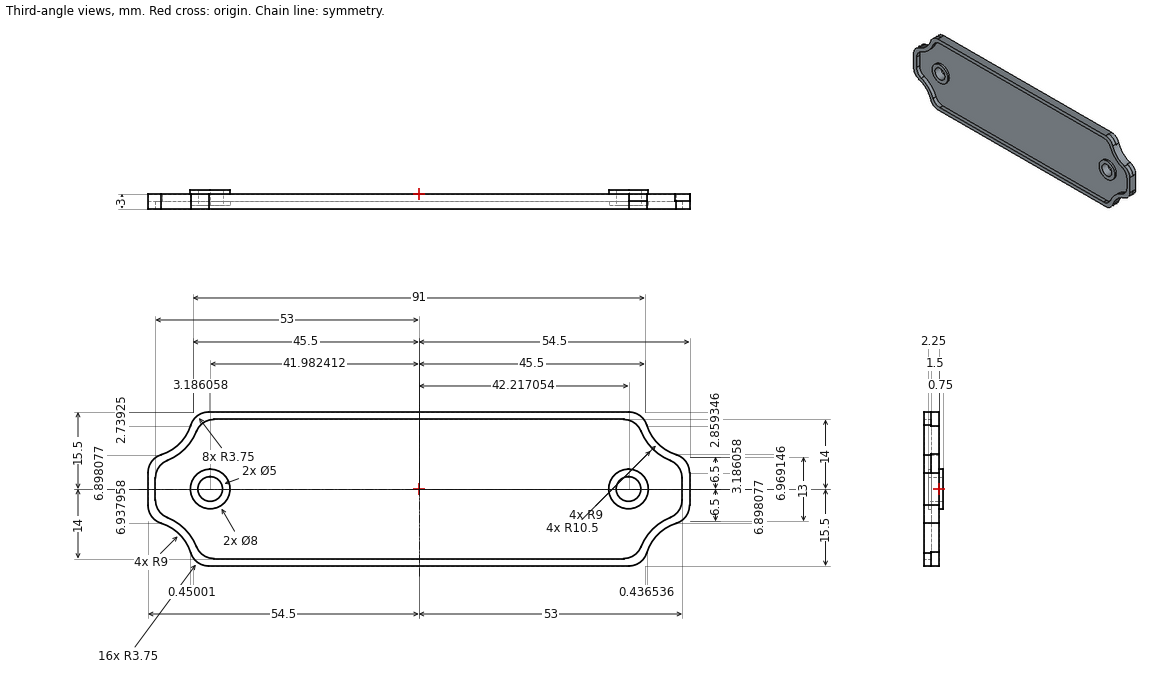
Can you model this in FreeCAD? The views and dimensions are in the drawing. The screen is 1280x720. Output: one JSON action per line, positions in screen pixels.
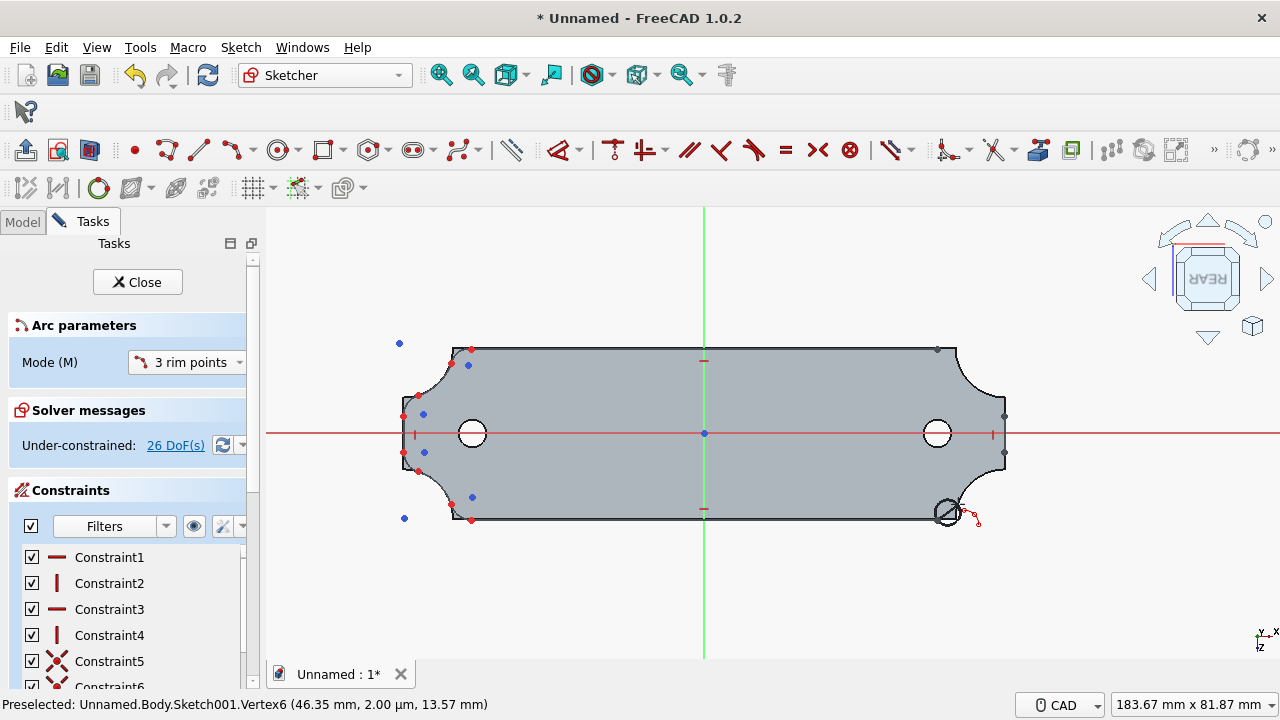
{"action": "scroll", "coordinate": [950, 515], "scroll_direction": "up", "scroll_amount": 7}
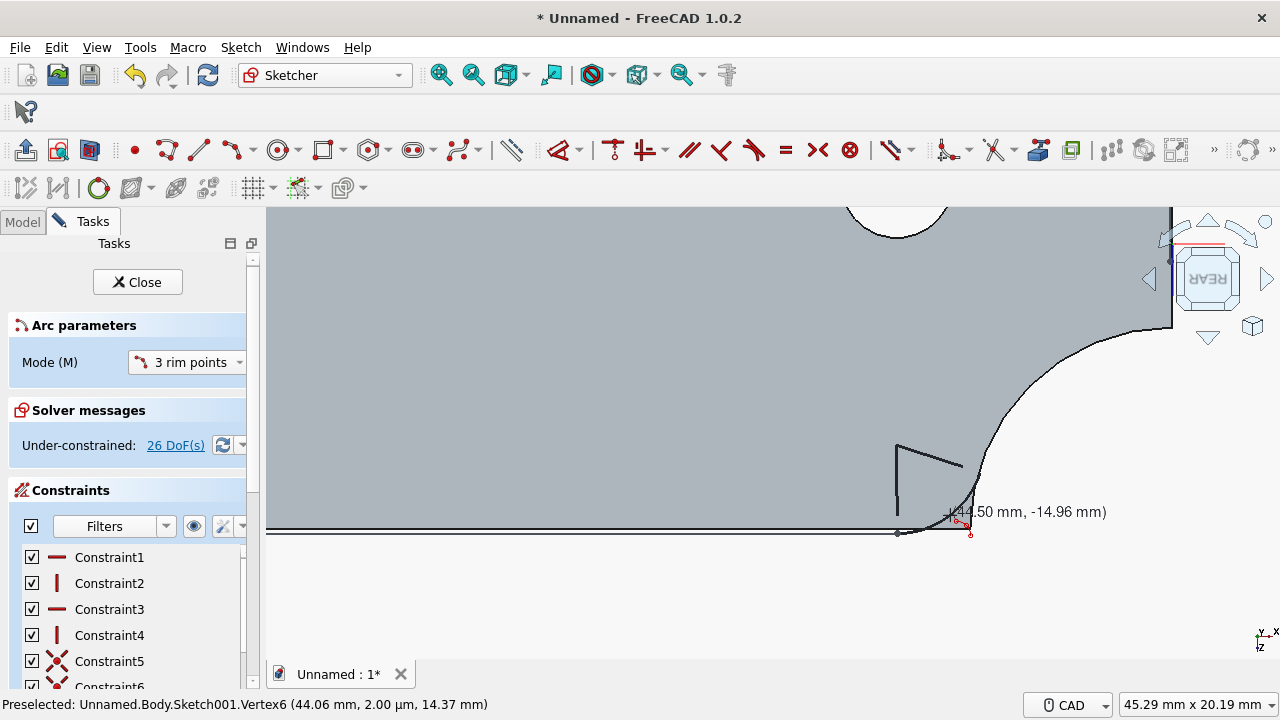
{"action": "left_click", "coordinate": [949, 513]}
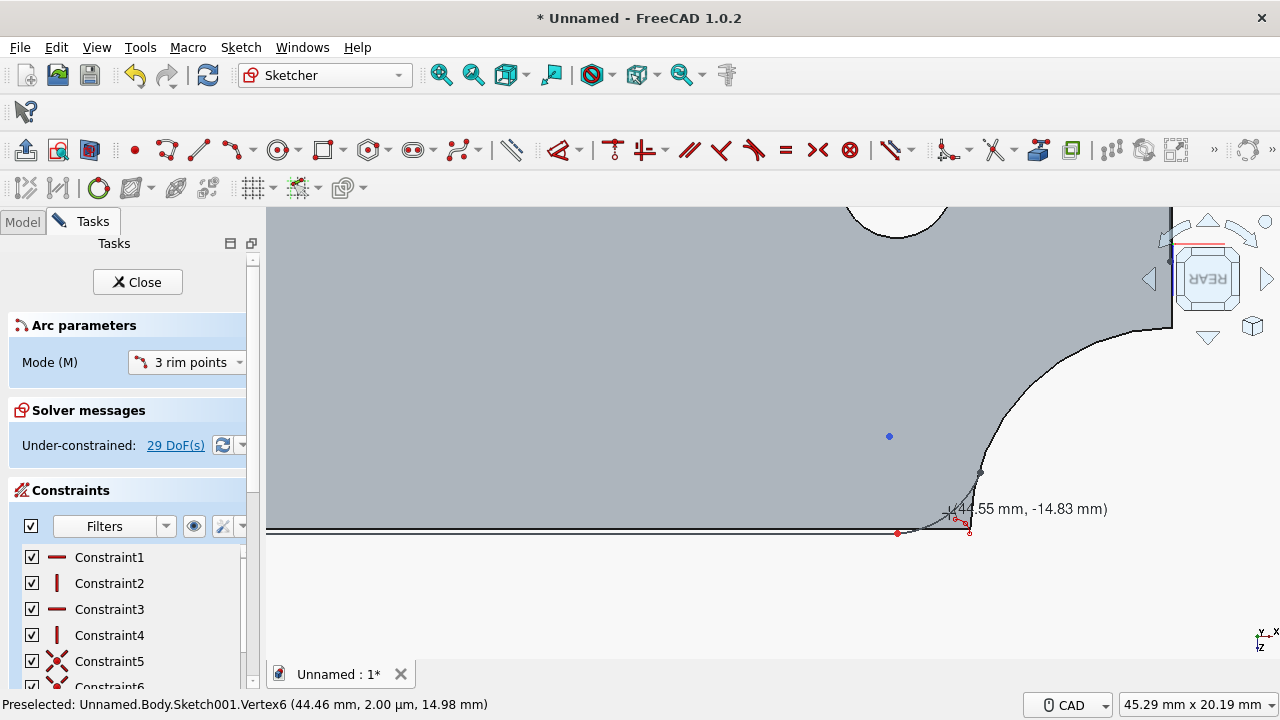
{"action": "scroll", "coordinate": [951, 515], "scroll_direction": "down", "scroll_amount": 7}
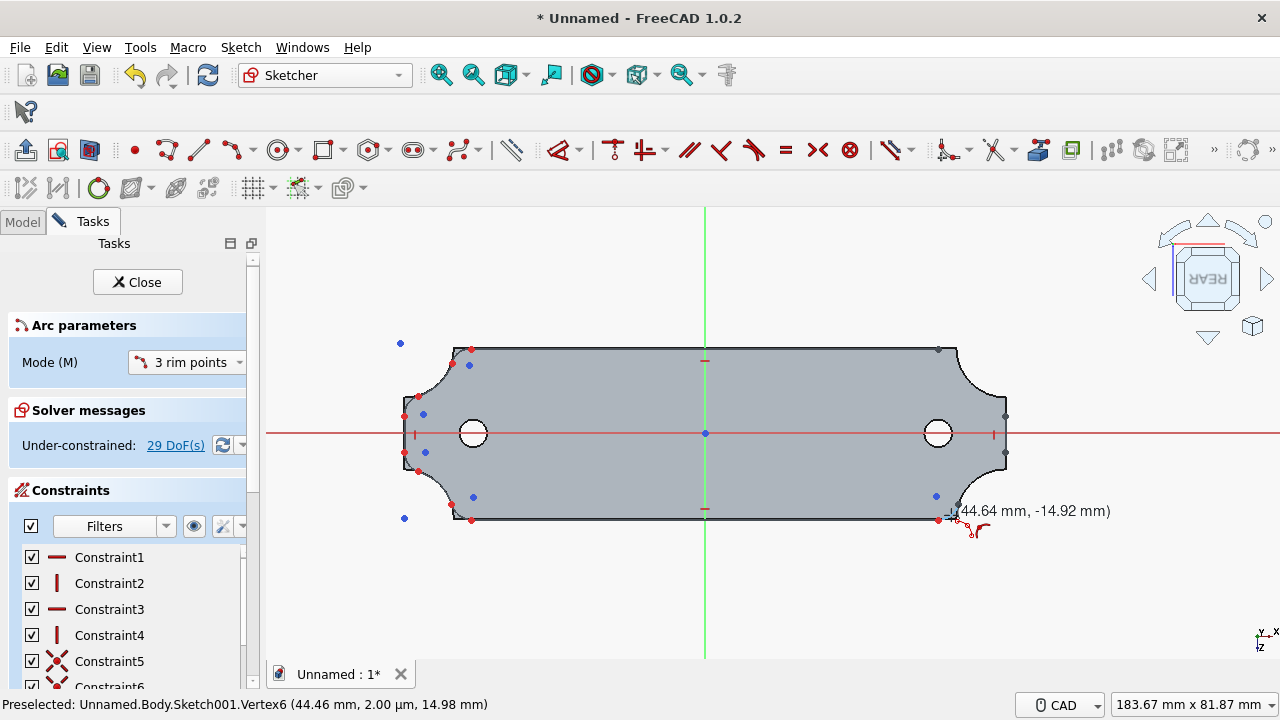
{"action": "left_click", "coordinate": [959, 505]}
{"action": "left_click", "coordinate": [991, 471]}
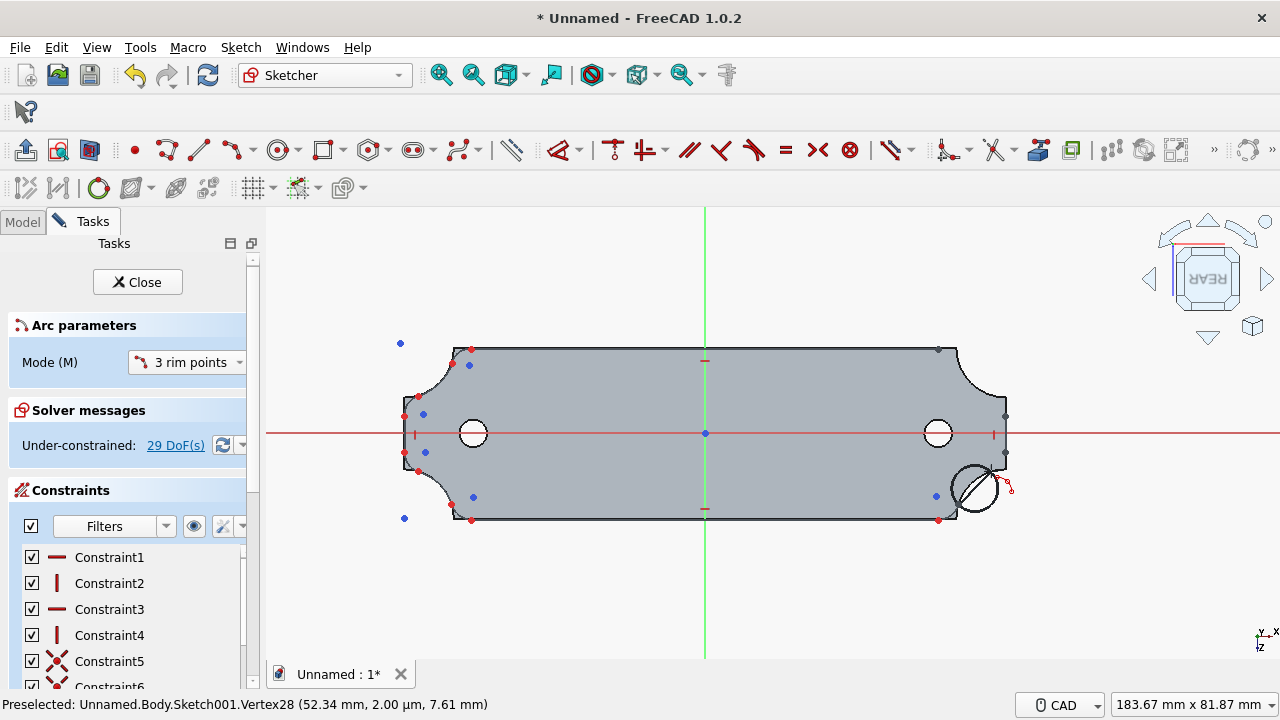
{"action": "scroll", "coordinate": [971, 484], "scroll_direction": "up", "scroll_amount": 6}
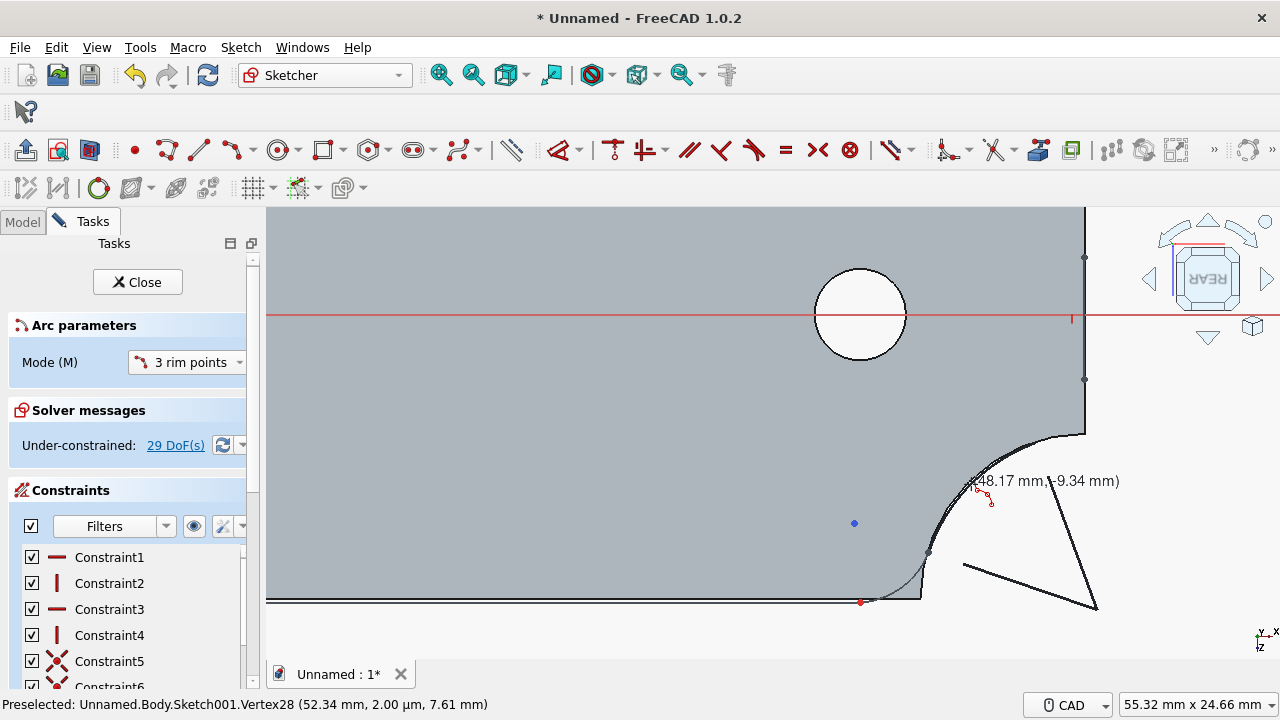
{"action": "left_click", "coordinate": [969, 482]}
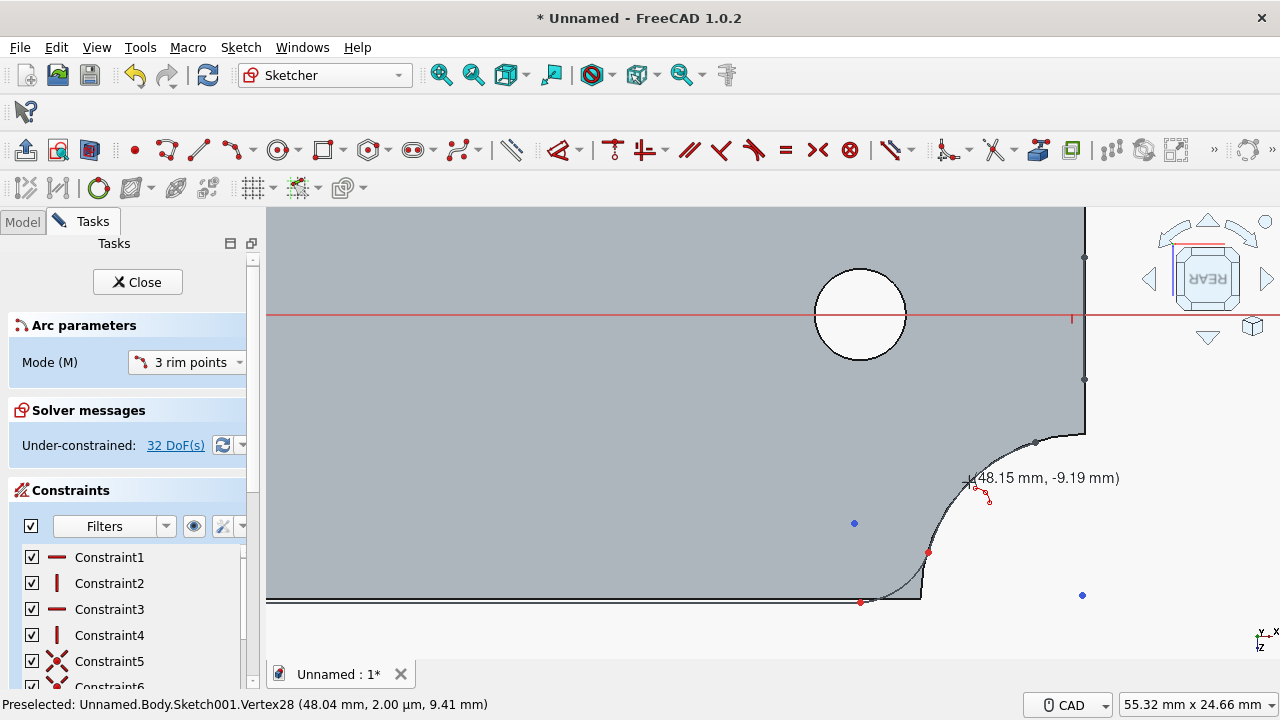
{"action": "scroll", "coordinate": [971, 484], "scroll_direction": "down", "scroll_amount": 6}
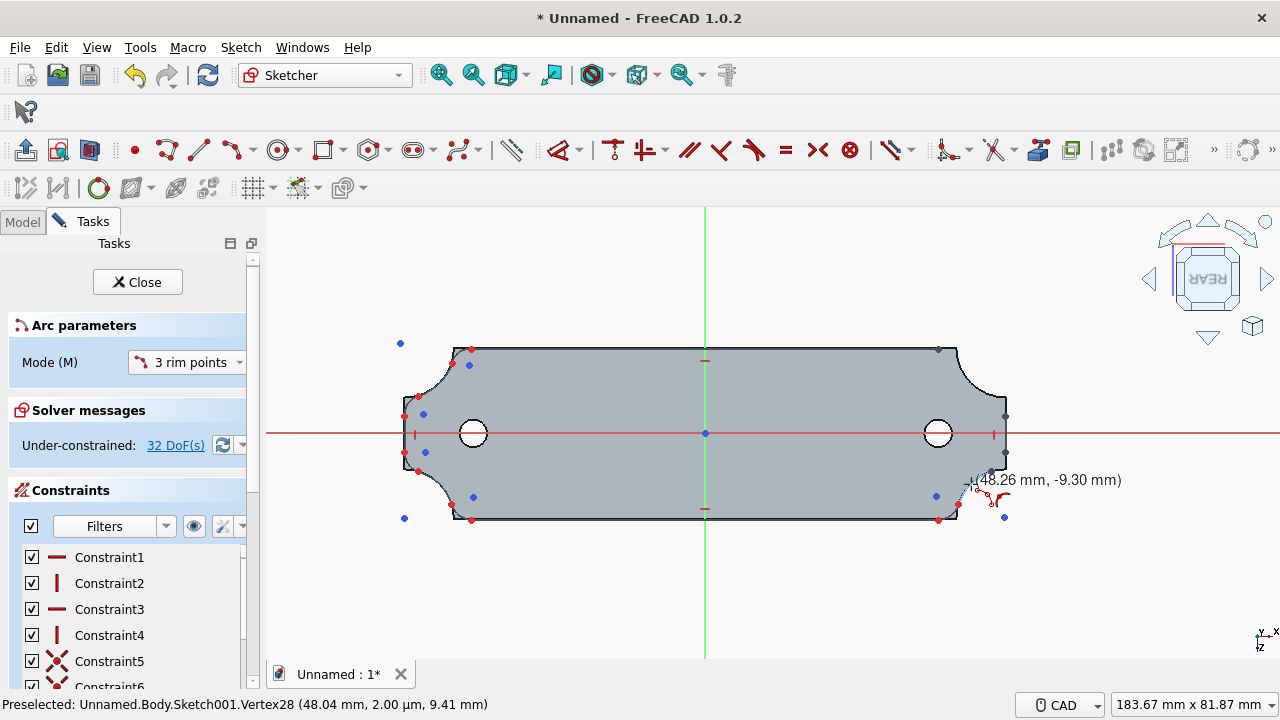
{"action": "left_click", "coordinate": [991, 472]}
{"action": "left_click", "coordinate": [1006, 453]}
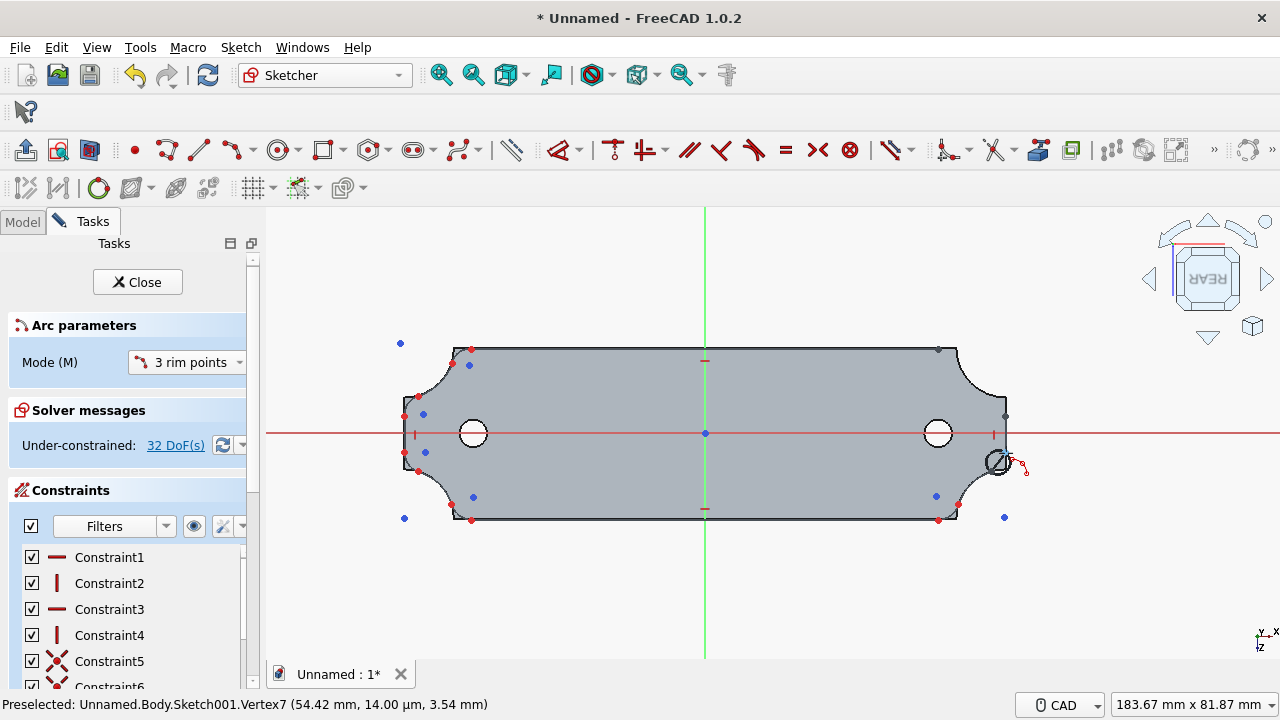
{"action": "scroll", "coordinate": [1002, 464], "scroll_direction": "up", "scroll_amount": 7}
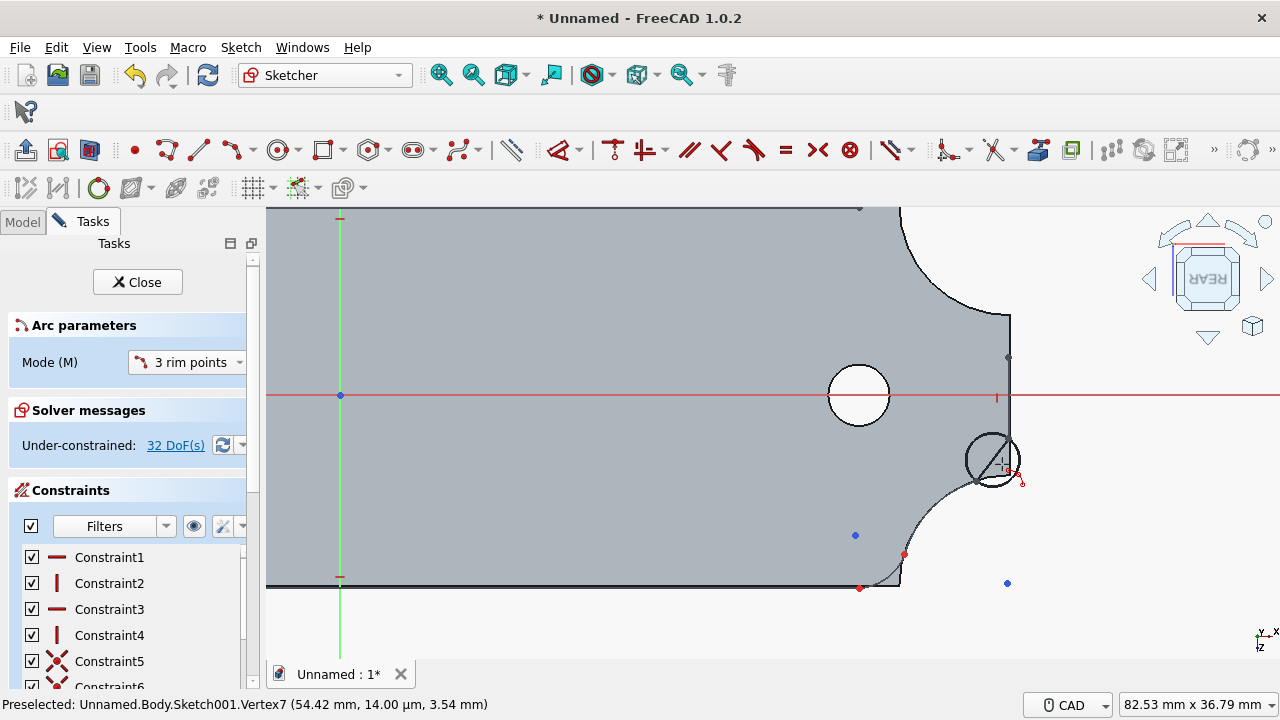
{"action": "left_click", "coordinate": [999, 462]}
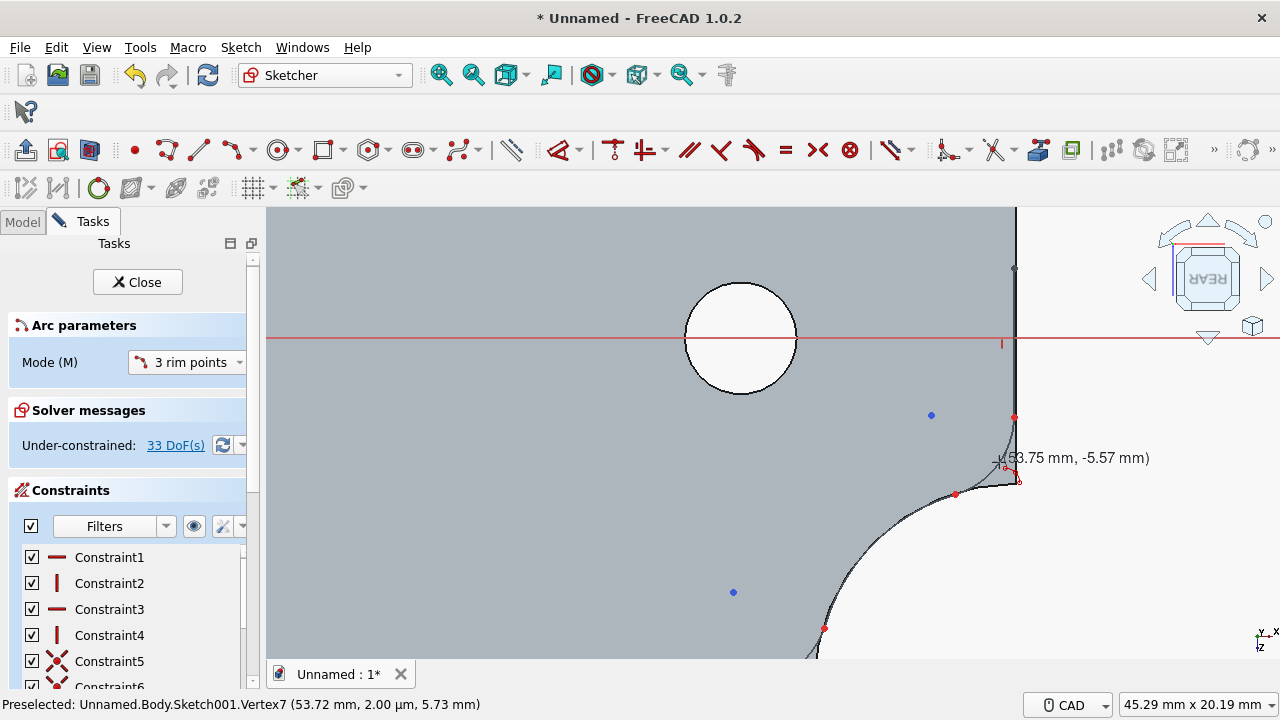
{"action": "scroll", "coordinate": [1002, 464], "scroll_direction": "down", "scroll_amount": 7}